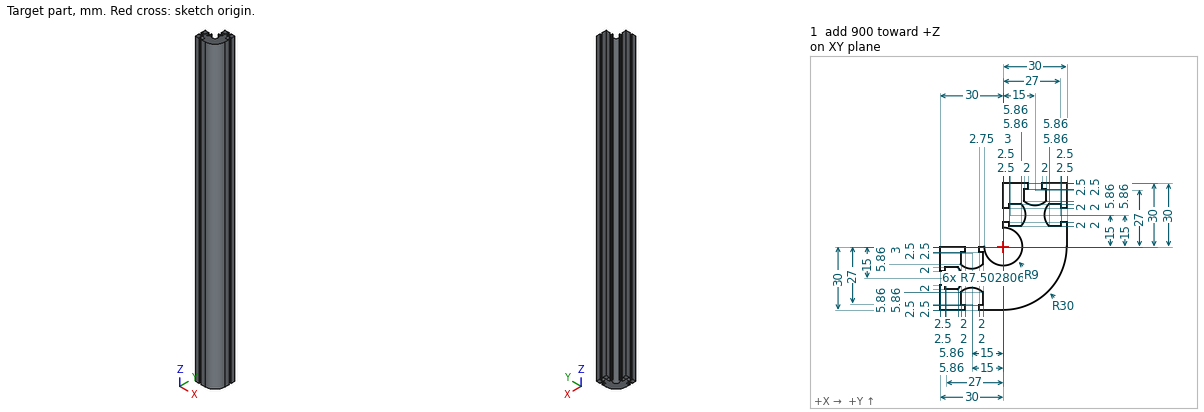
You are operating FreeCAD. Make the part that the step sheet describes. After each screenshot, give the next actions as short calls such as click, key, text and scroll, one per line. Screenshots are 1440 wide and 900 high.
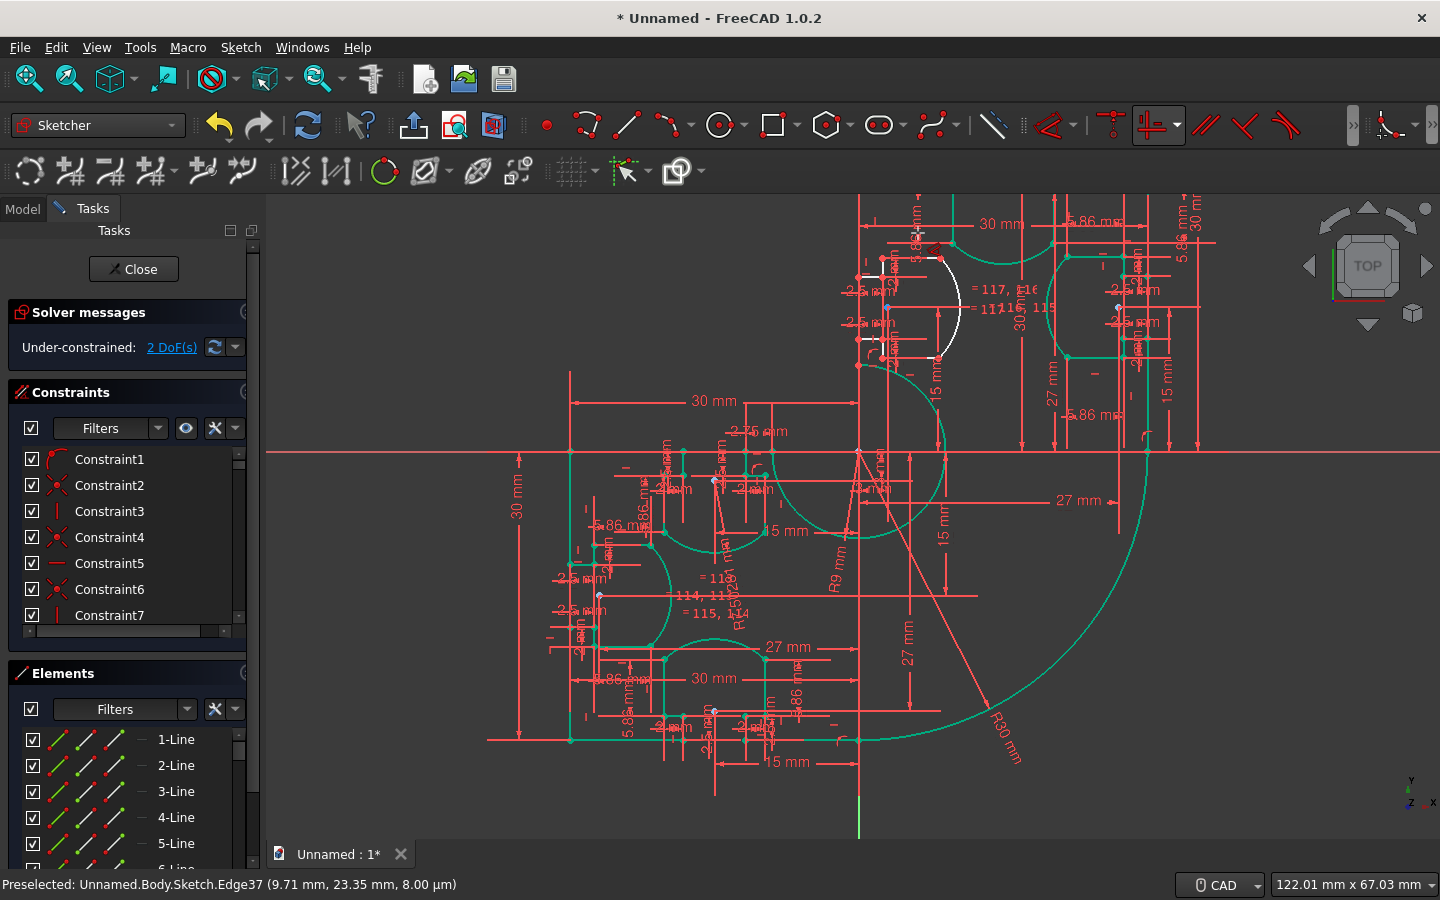
click(900, 258)
click(912, 412)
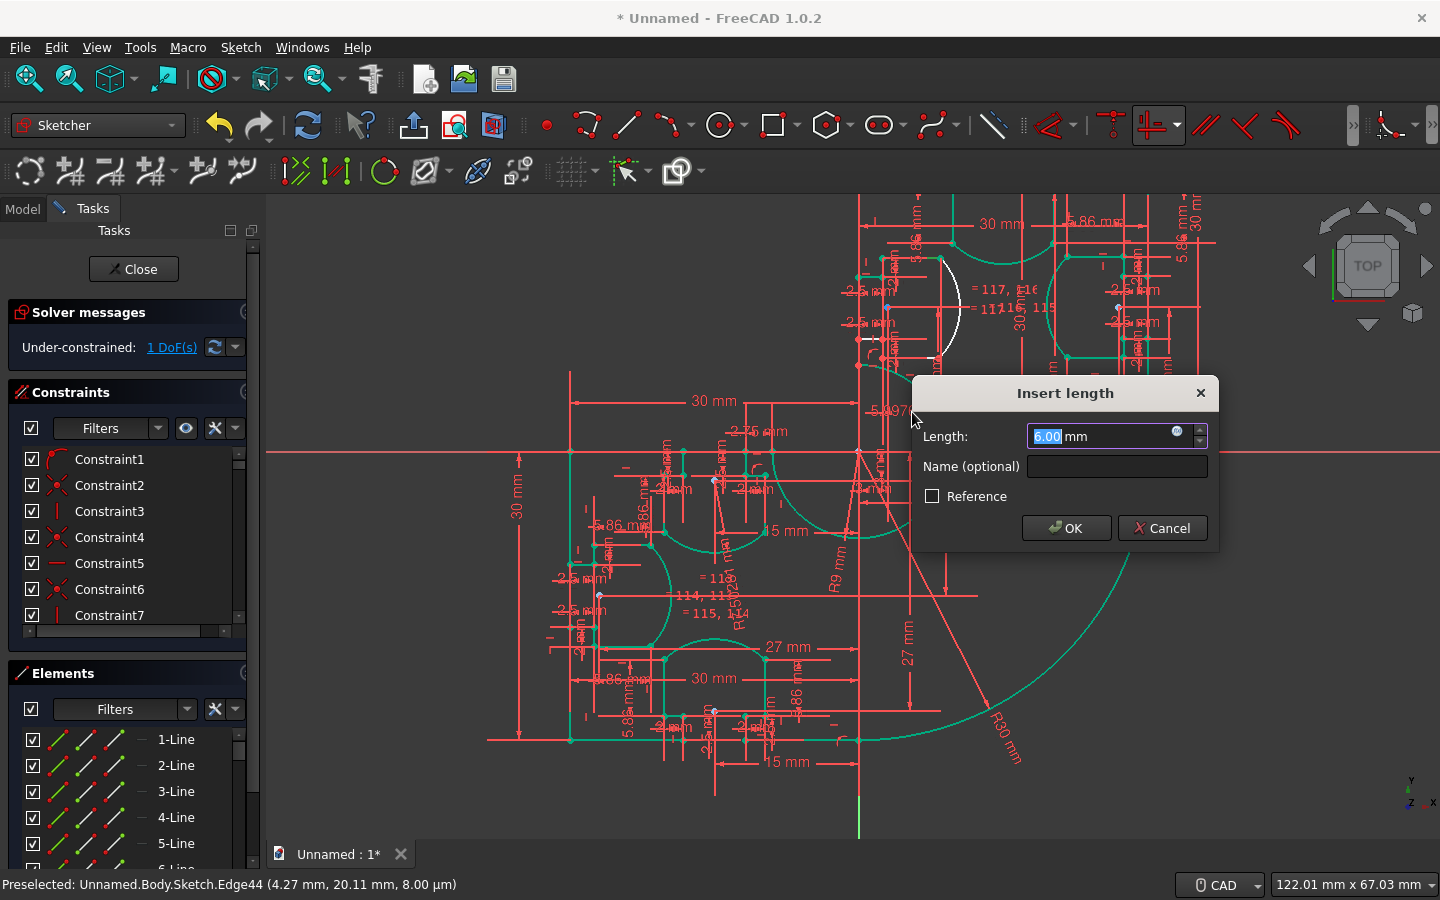
text(5.86)
key(Return)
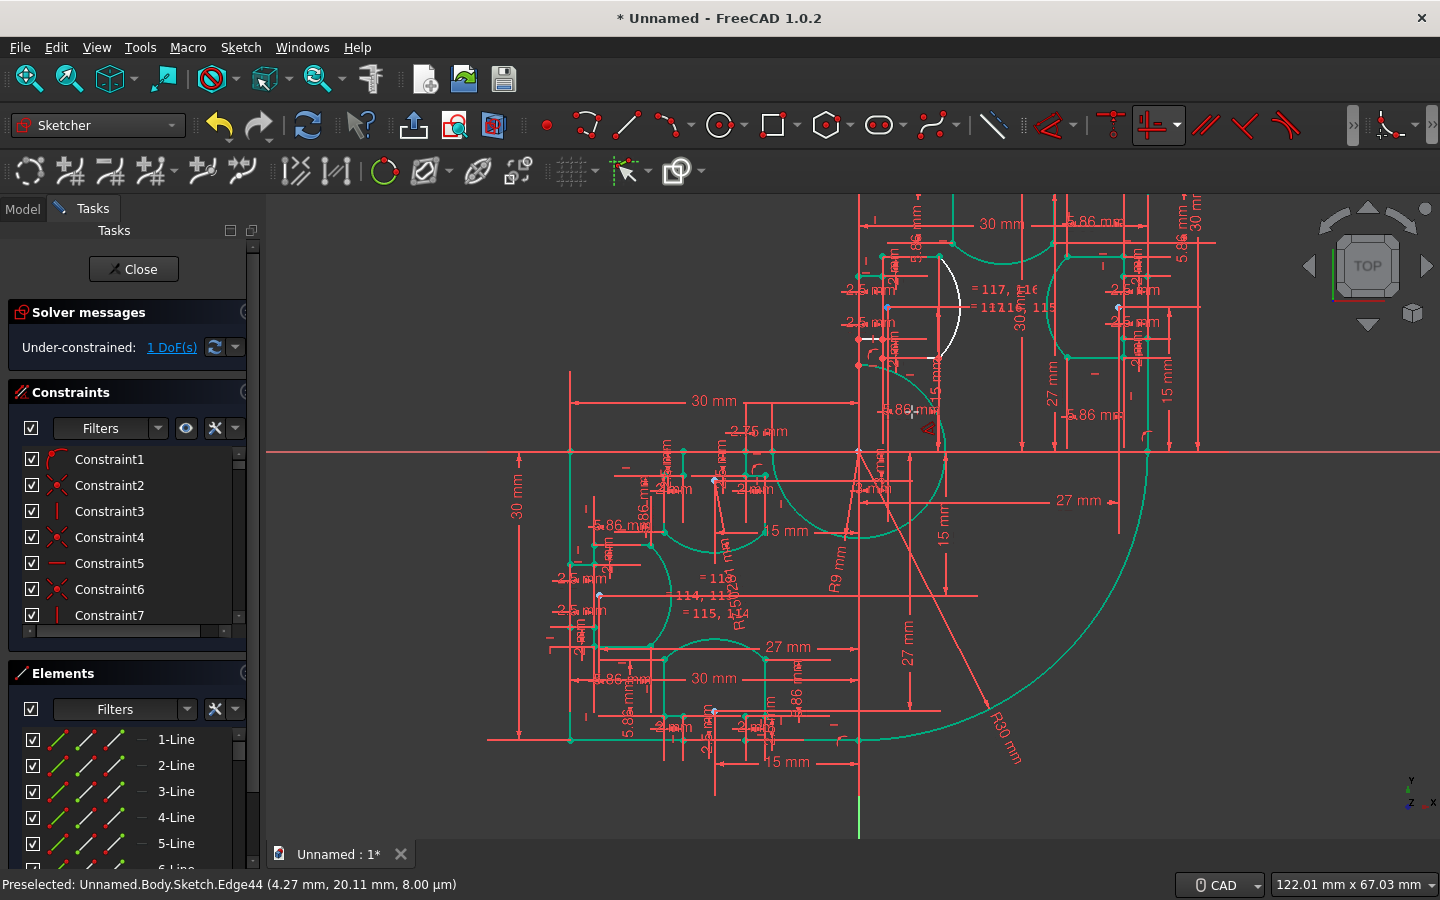
click(922, 358)
click(911, 324)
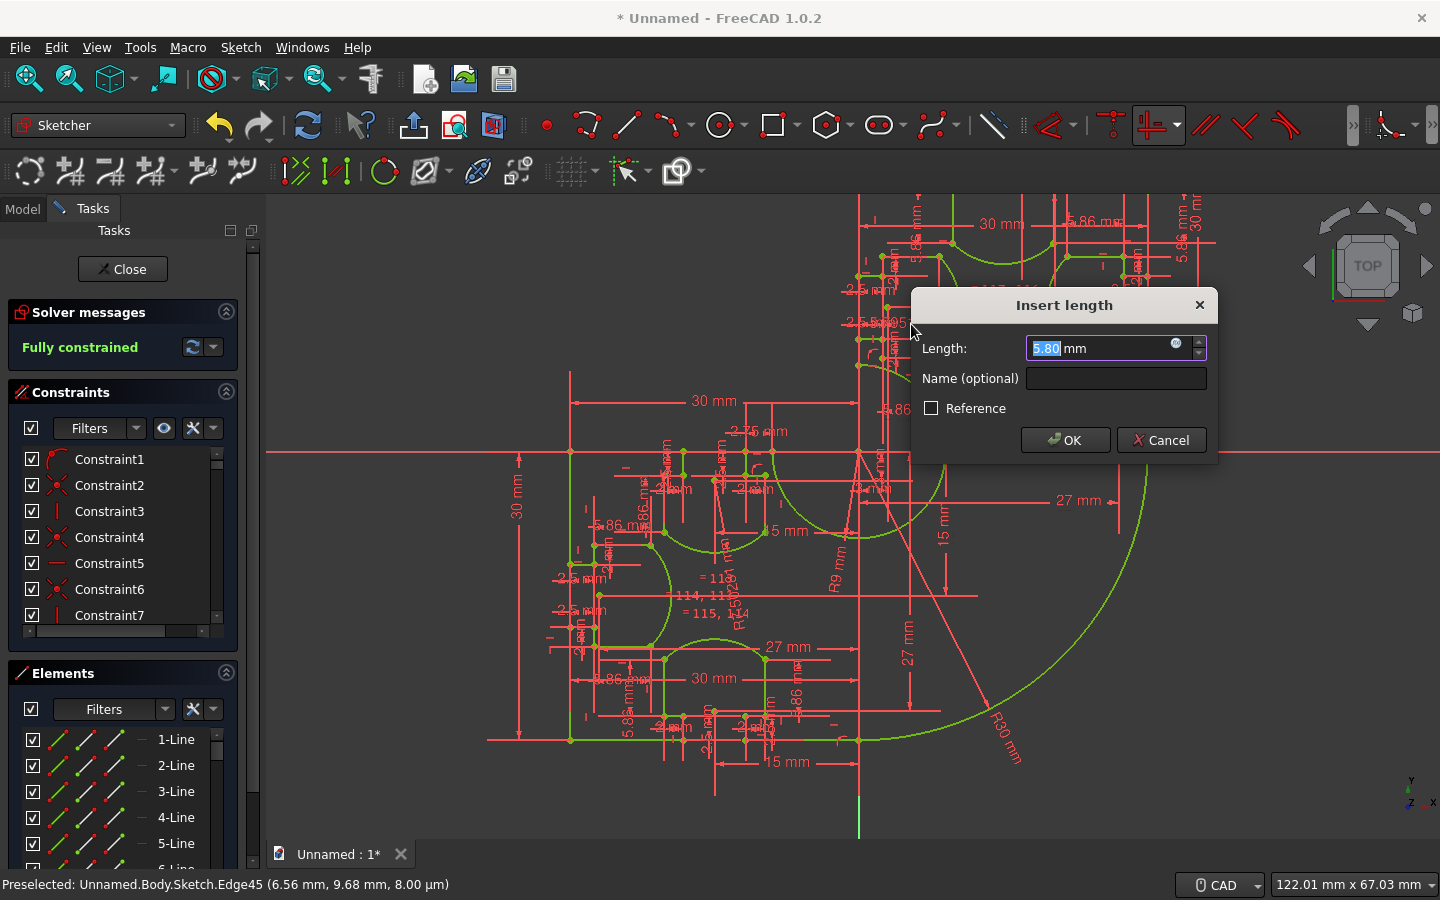
text(5.86)
key(Return)
key(Escape)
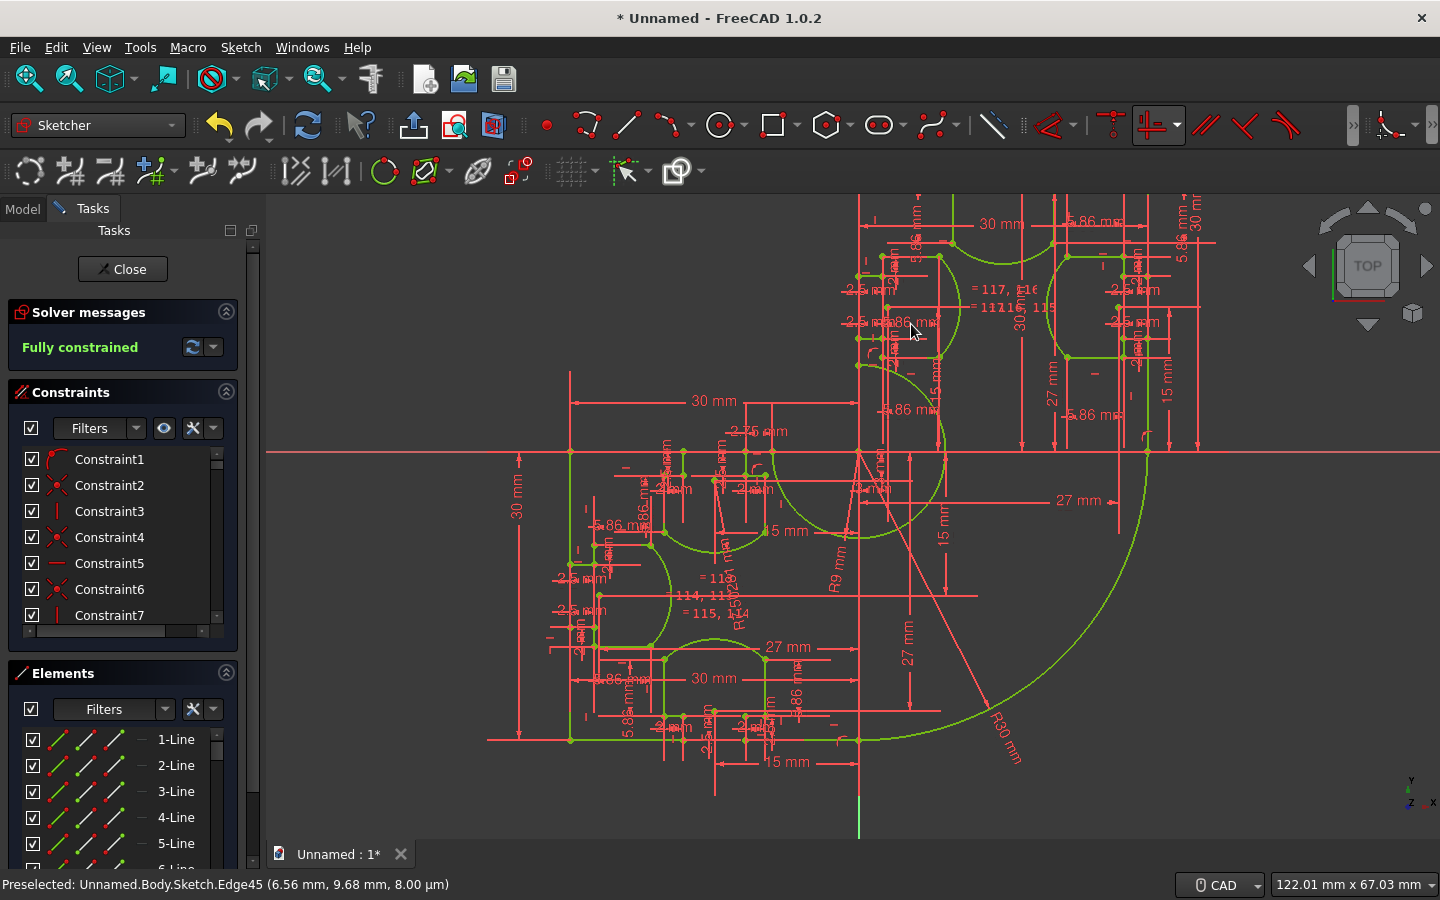
click(123, 269)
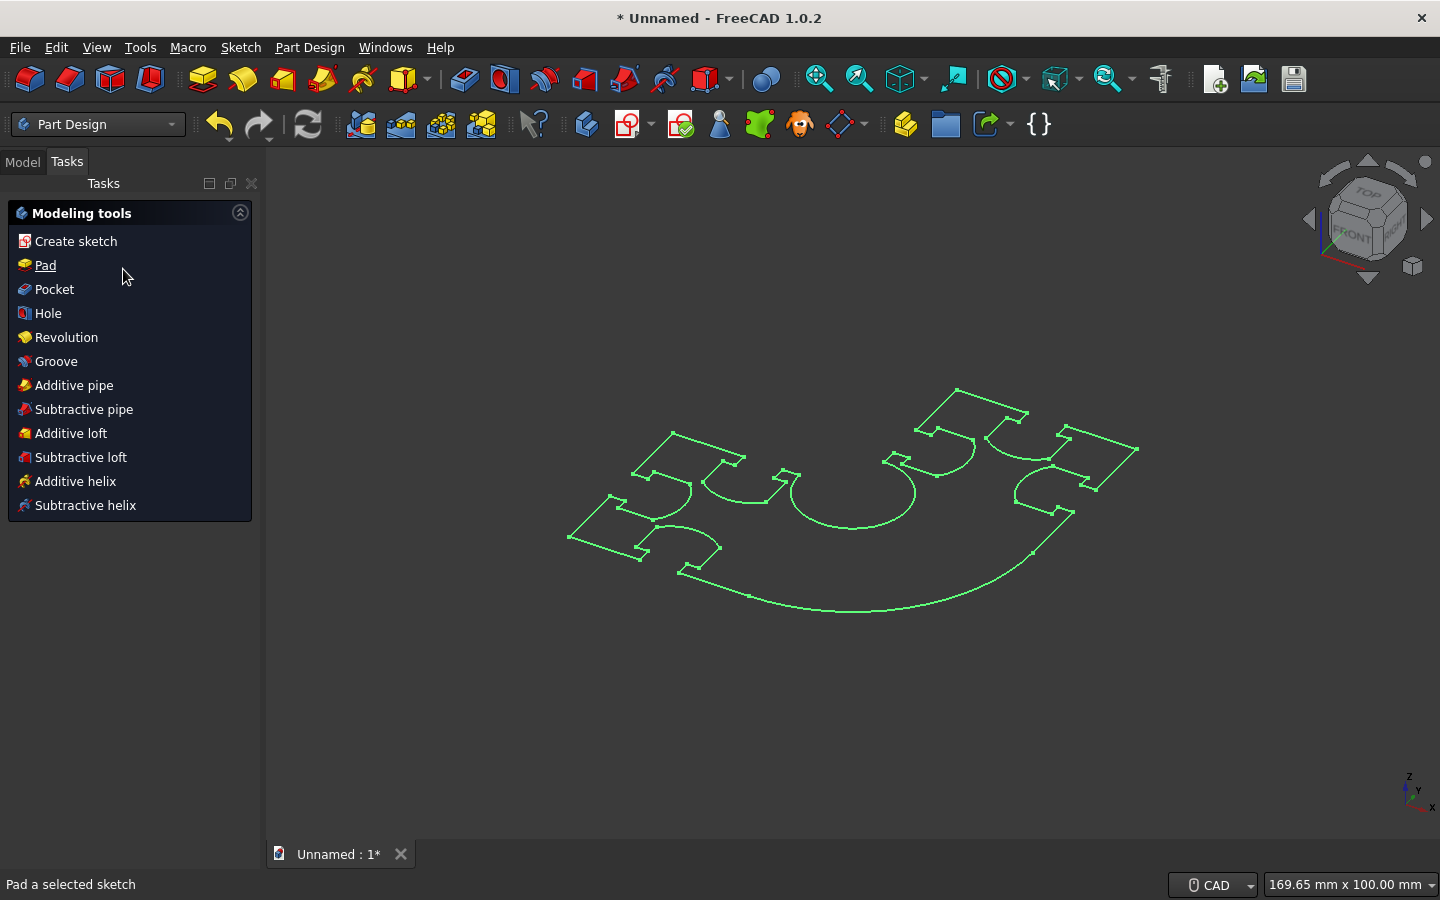
click(204, 80)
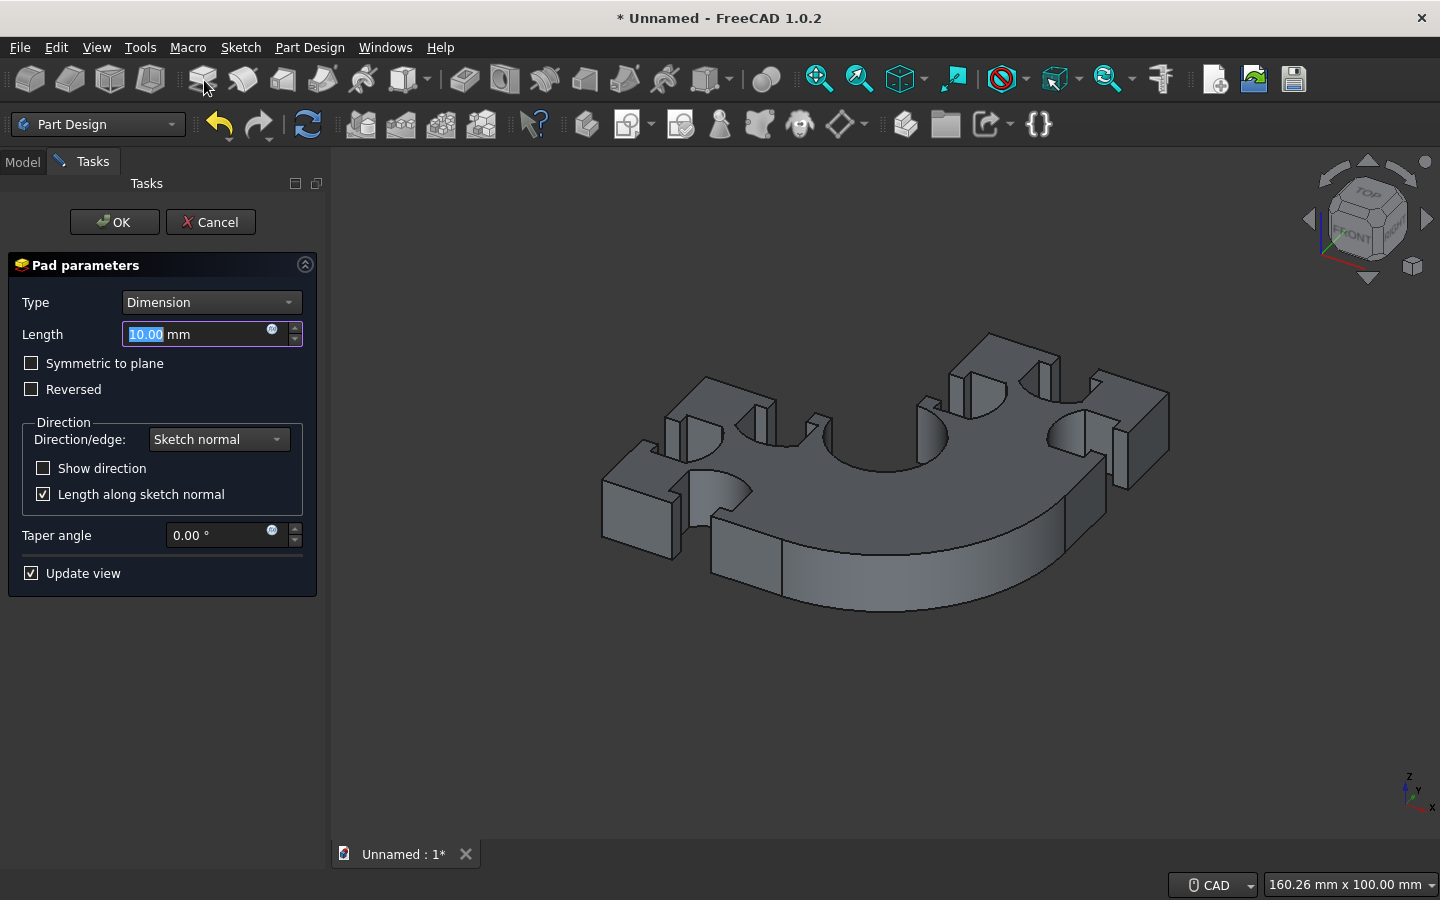
text(900)
key(Tab)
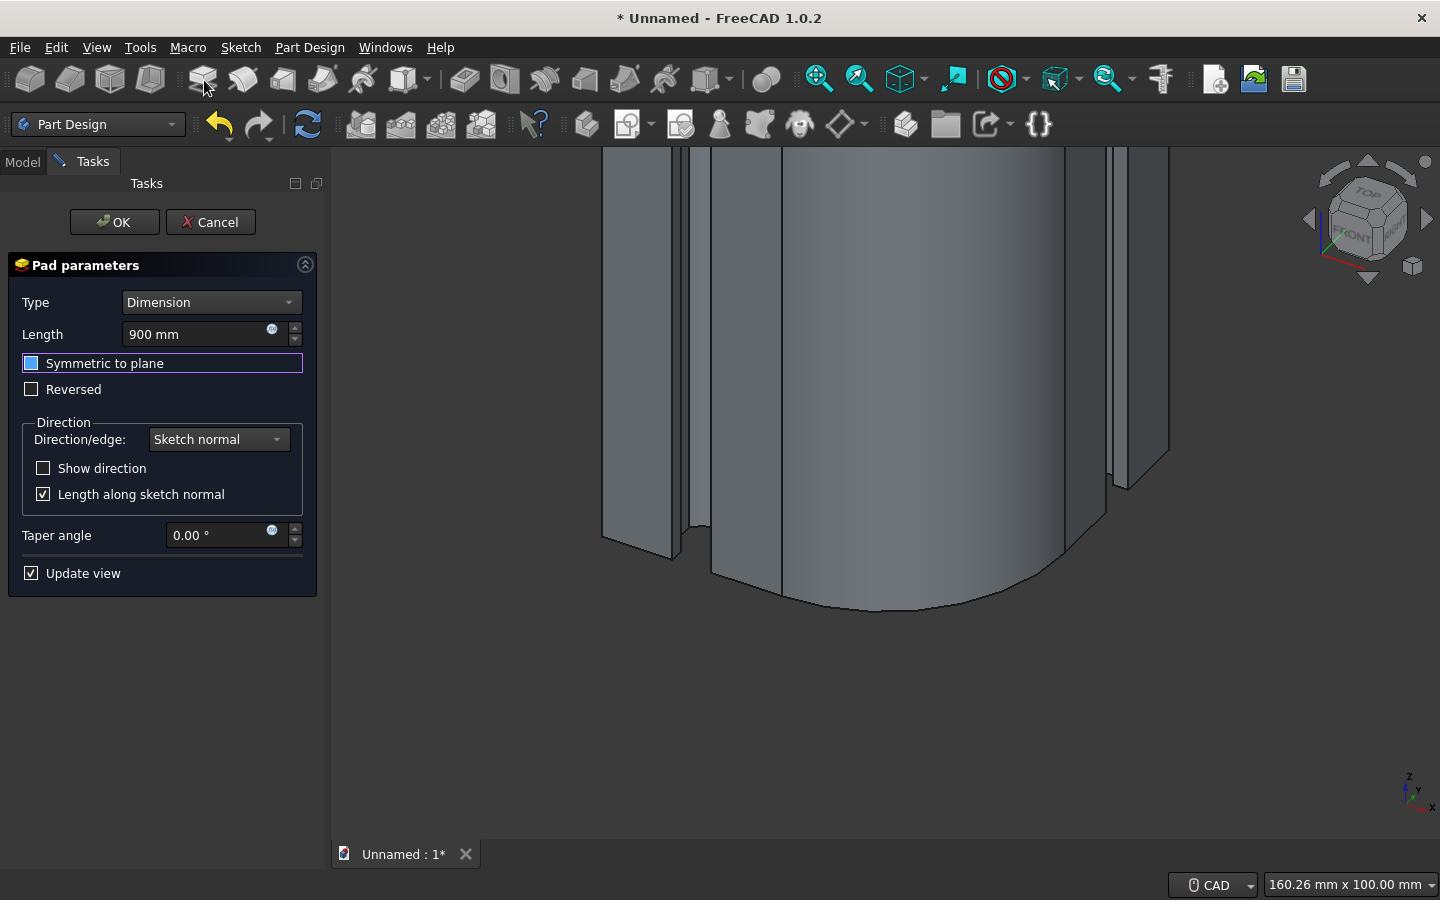
click(115, 222)